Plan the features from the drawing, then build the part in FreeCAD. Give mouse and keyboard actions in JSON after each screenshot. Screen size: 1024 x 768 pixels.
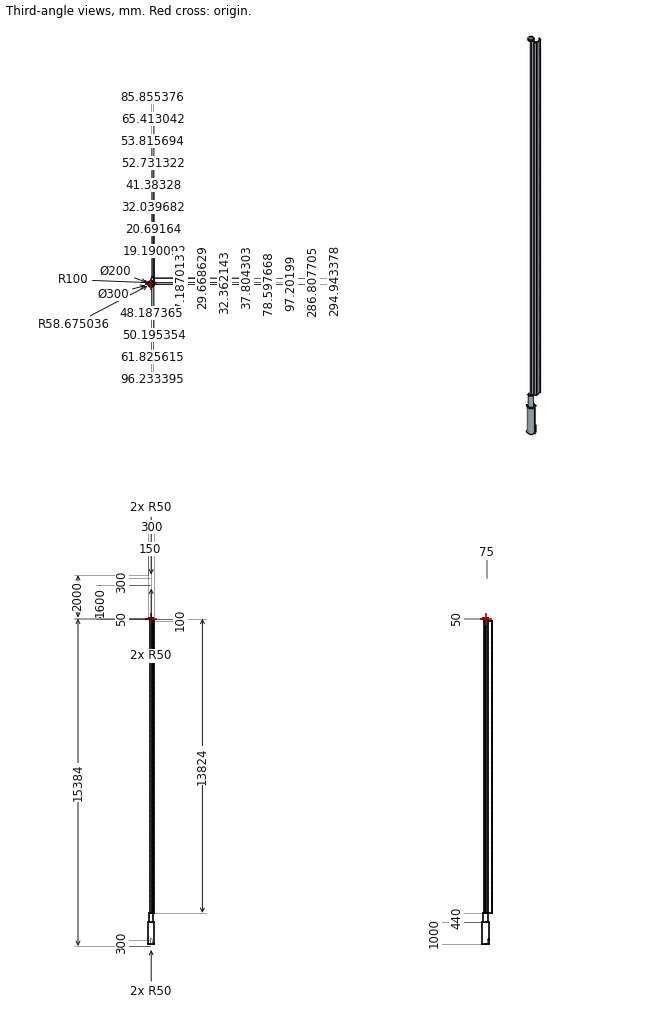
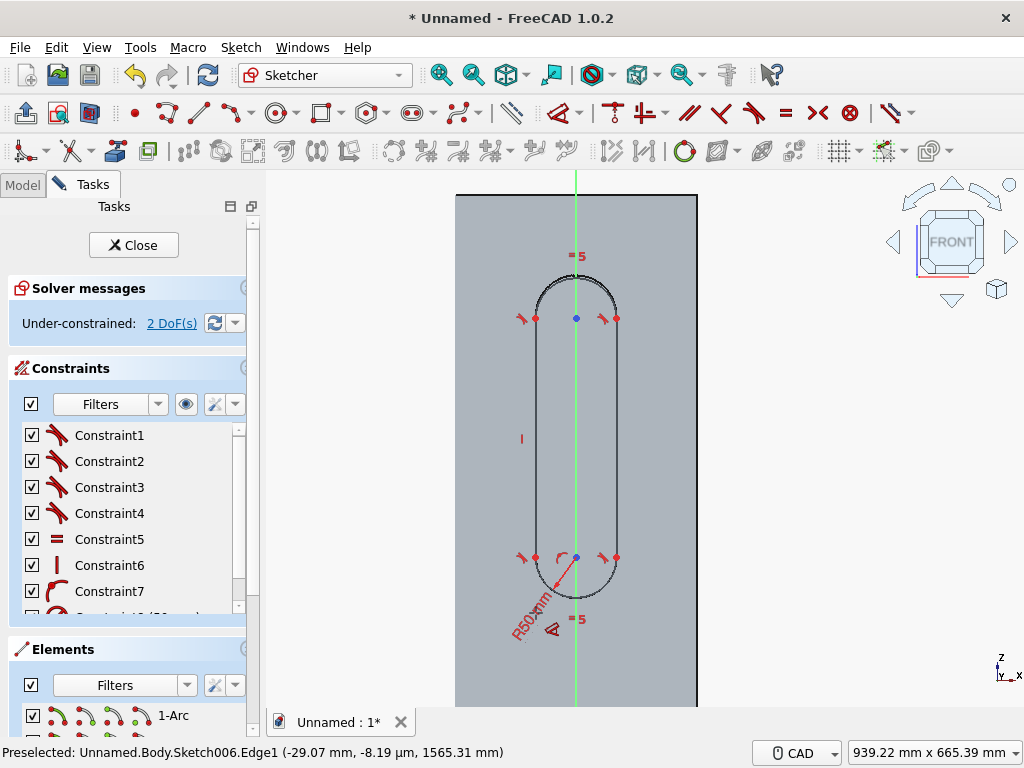
{"action": "left_click", "coordinate": [536, 486]}
{"action": "left_click", "coordinate": [502, 438]}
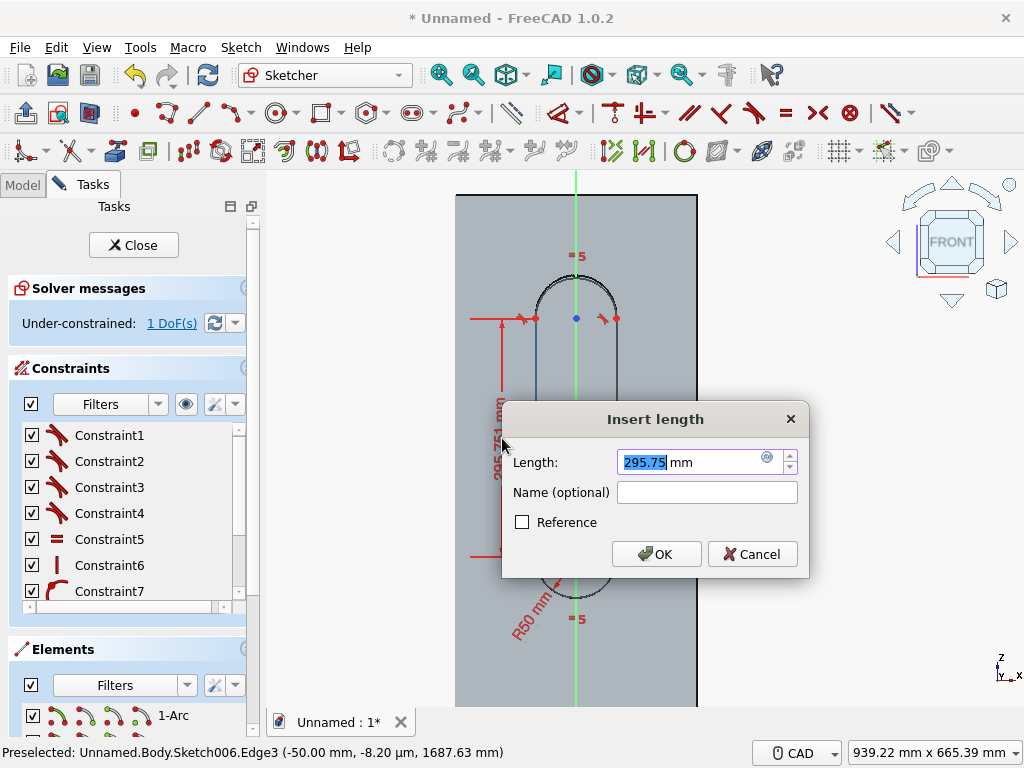
{"action": "type", "text": "300"}
{"action": "key", "text": "Return"}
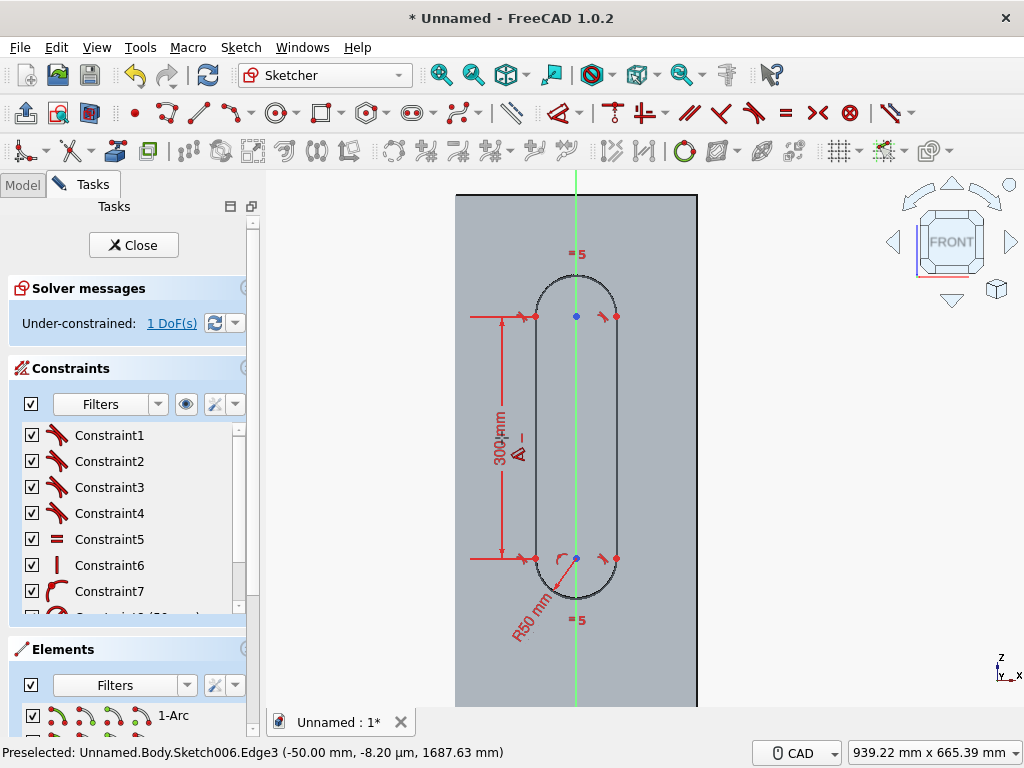
{"action": "left_click", "coordinate": [536, 559]}
{"action": "left_click", "coordinate": [502, 591]}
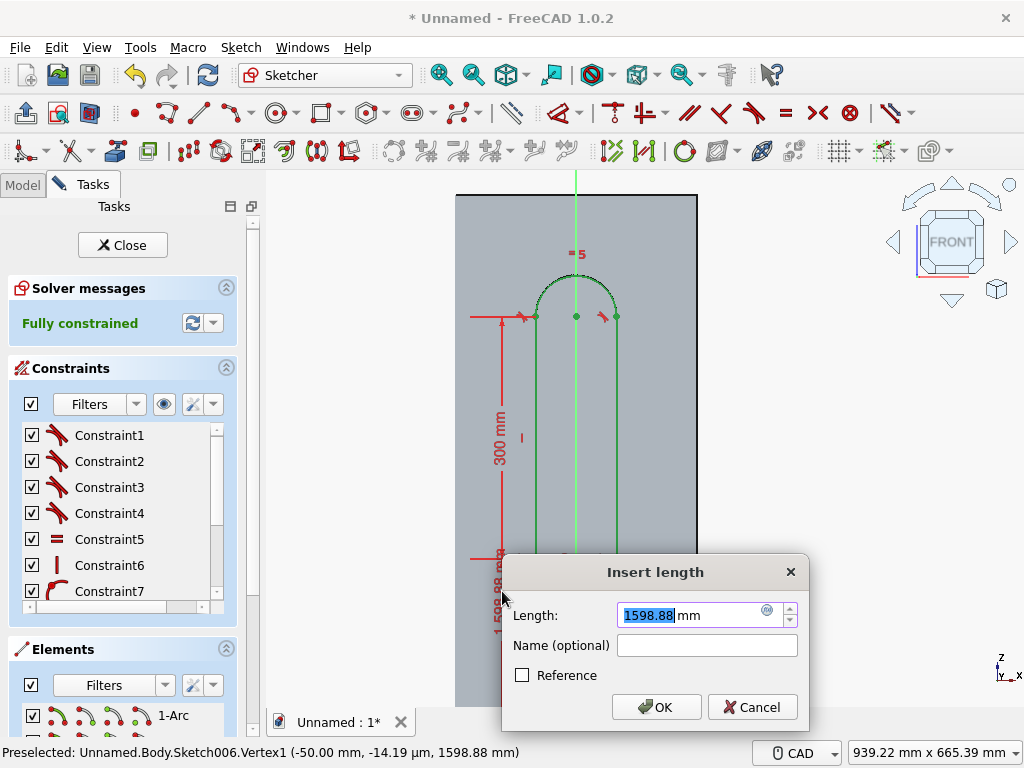
{"action": "type", "text": "1600"}
{"action": "key", "text": "Return"}
{"action": "key", "text": "Escape"}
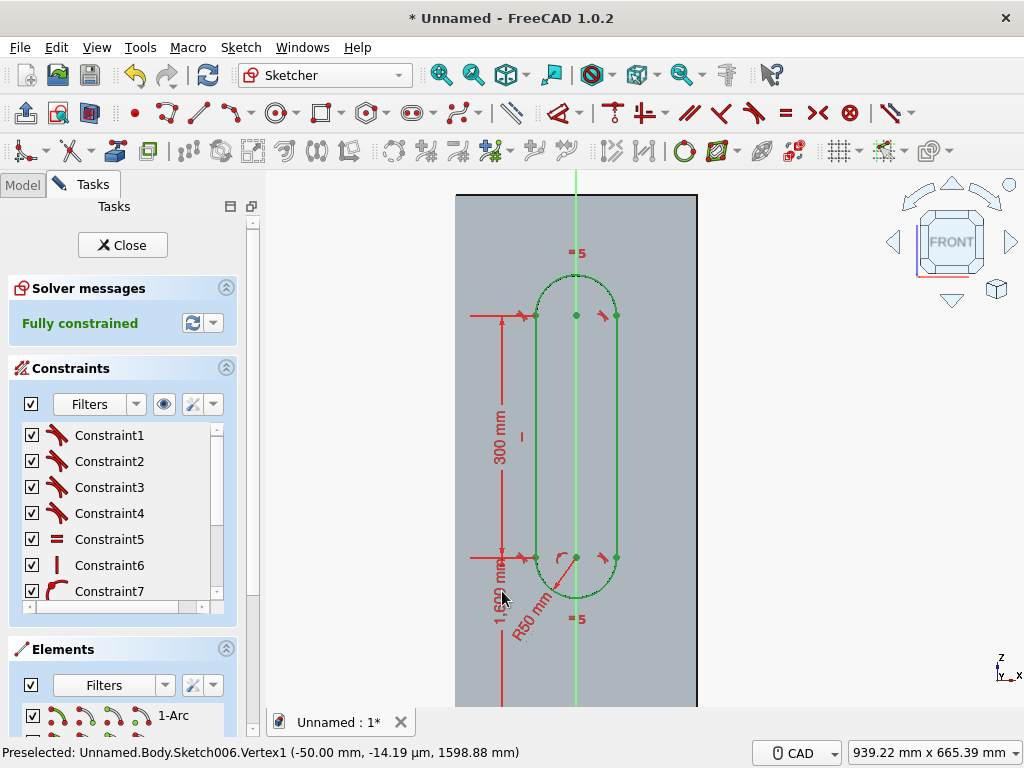
{"action": "left_click", "coordinate": [123, 245]}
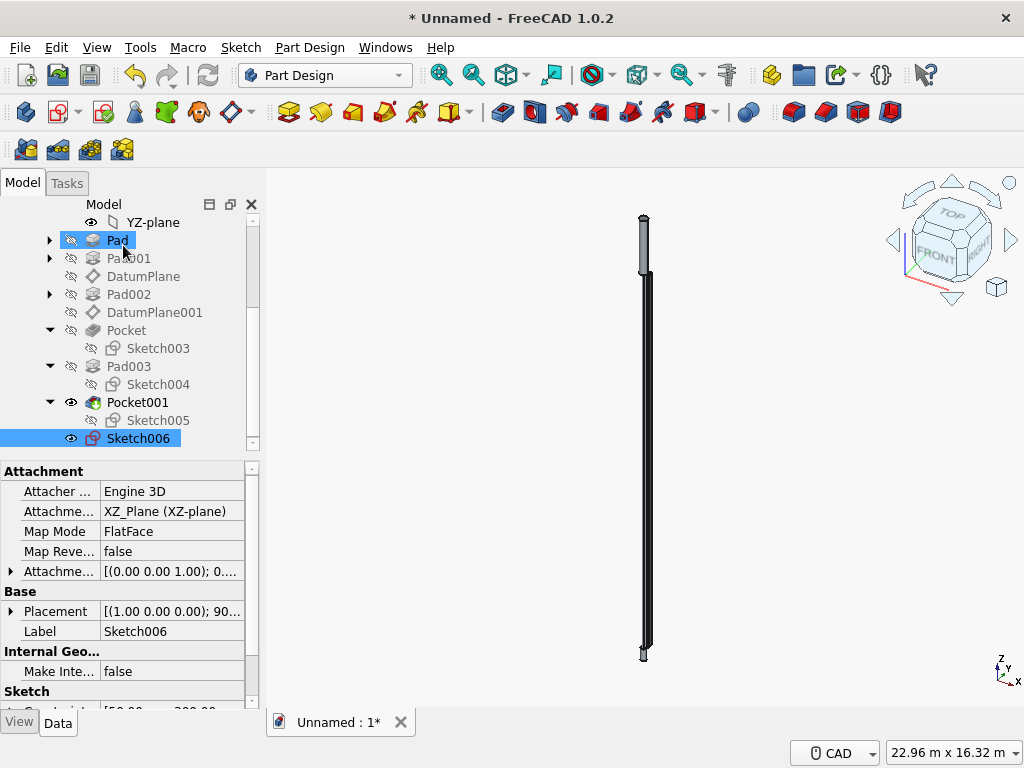
{"action": "left_click", "coordinate": [290, 112]}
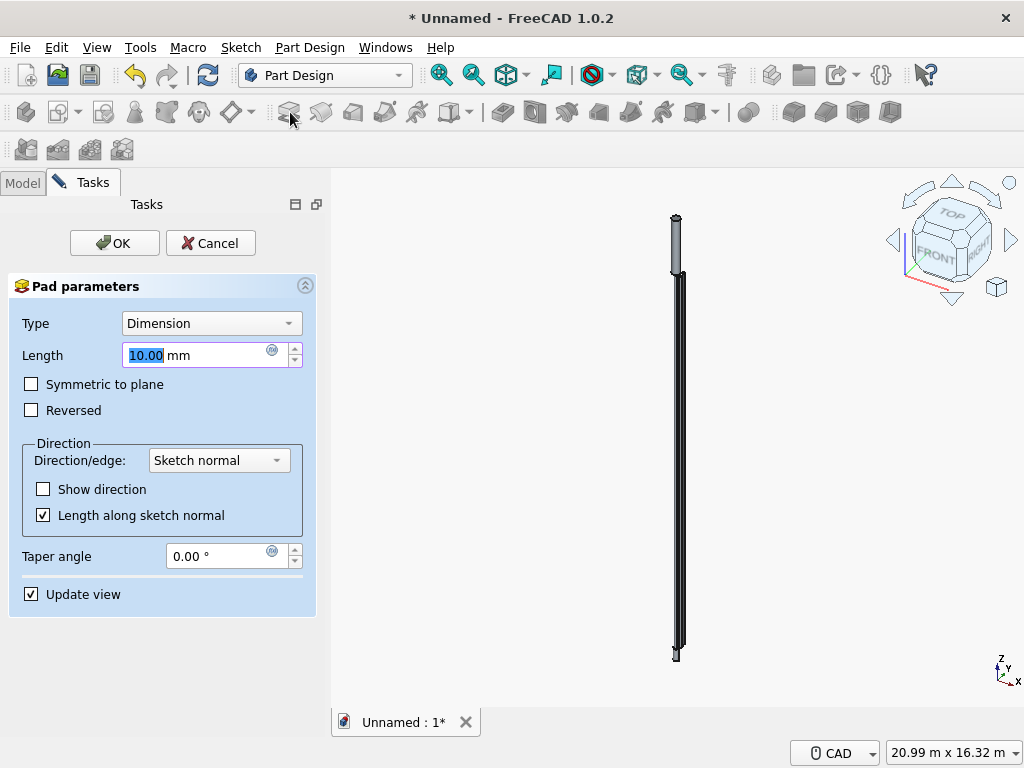
{"action": "type", "text": "75"}
{"action": "key", "text": "Tab"}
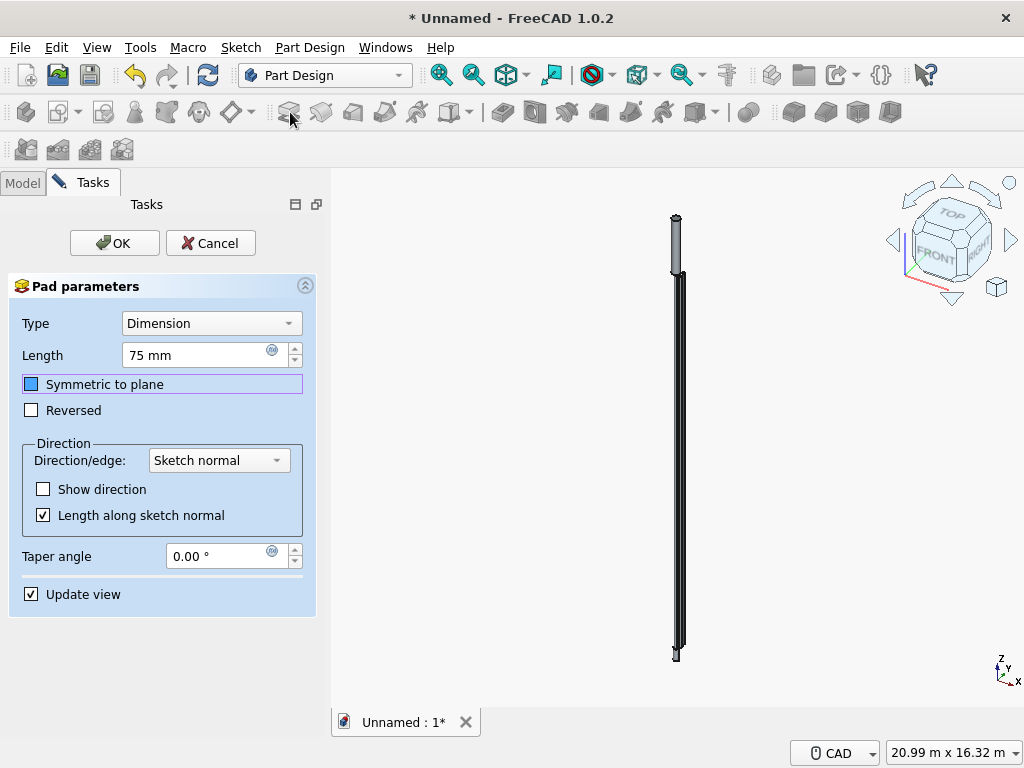
{"action": "left_click", "coordinate": [30, 410]}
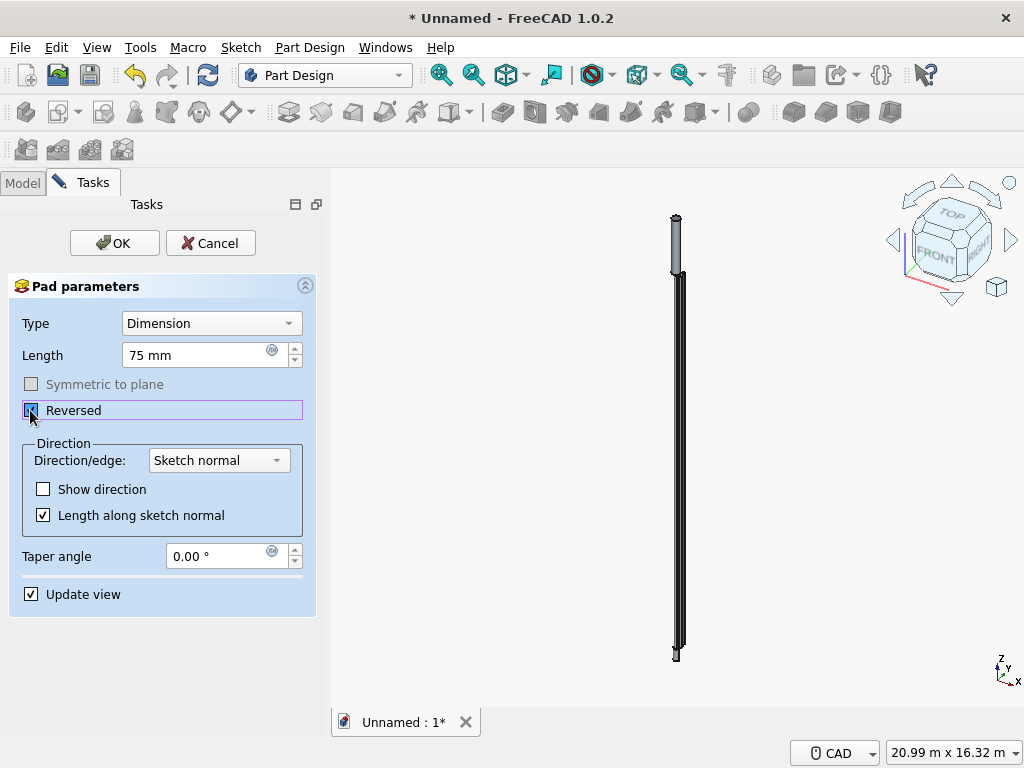
{"action": "left_click", "coordinate": [115, 243]}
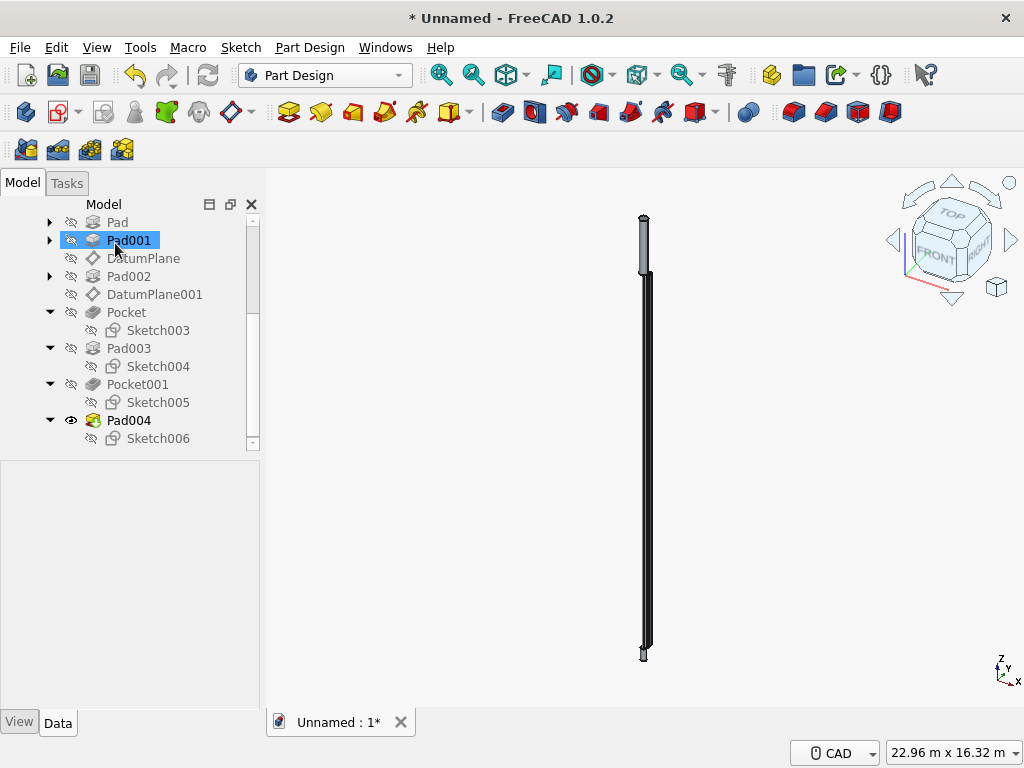
{"action": "scroll", "coordinate": [140, 326], "scroll_direction": "down", "scroll_amount": 3}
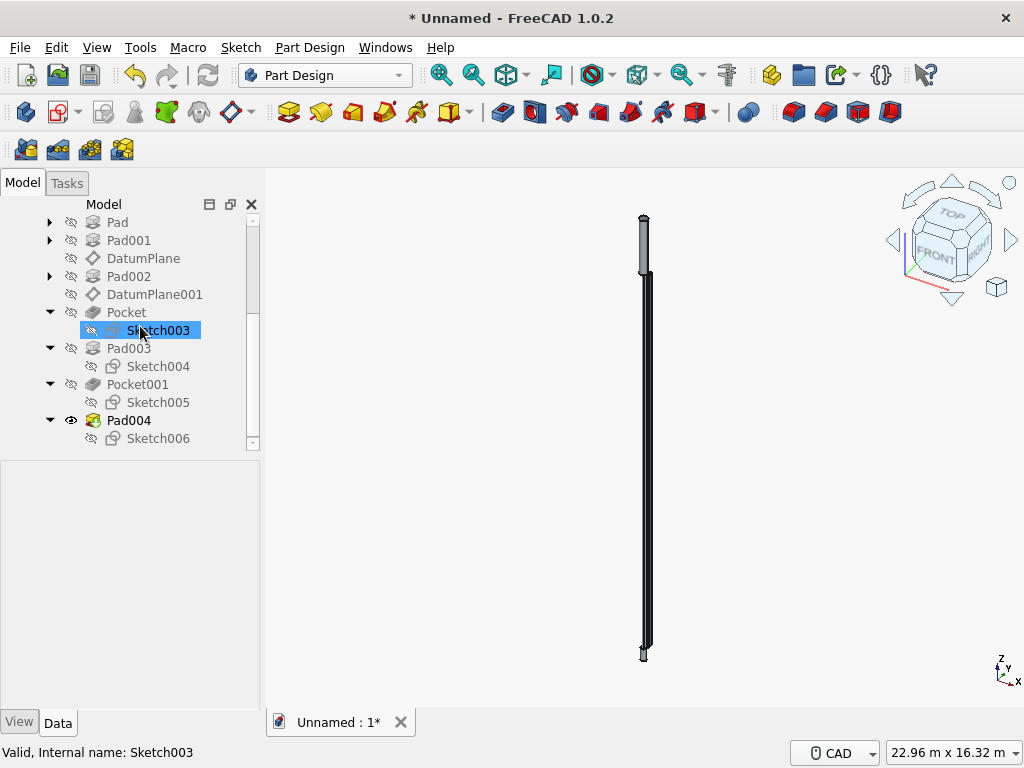
{"action": "scroll", "coordinate": [140, 326], "scroll_direction": "up", "scroll_amount": 15}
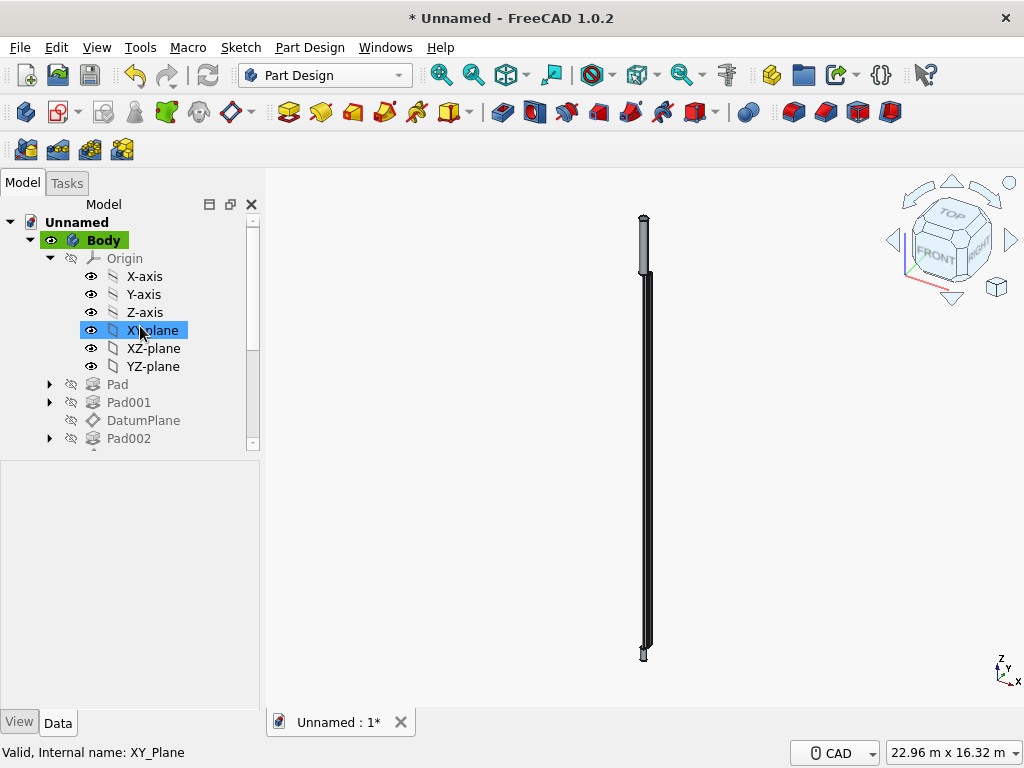
{"action": "left_click", "coordinate": [136, 330]}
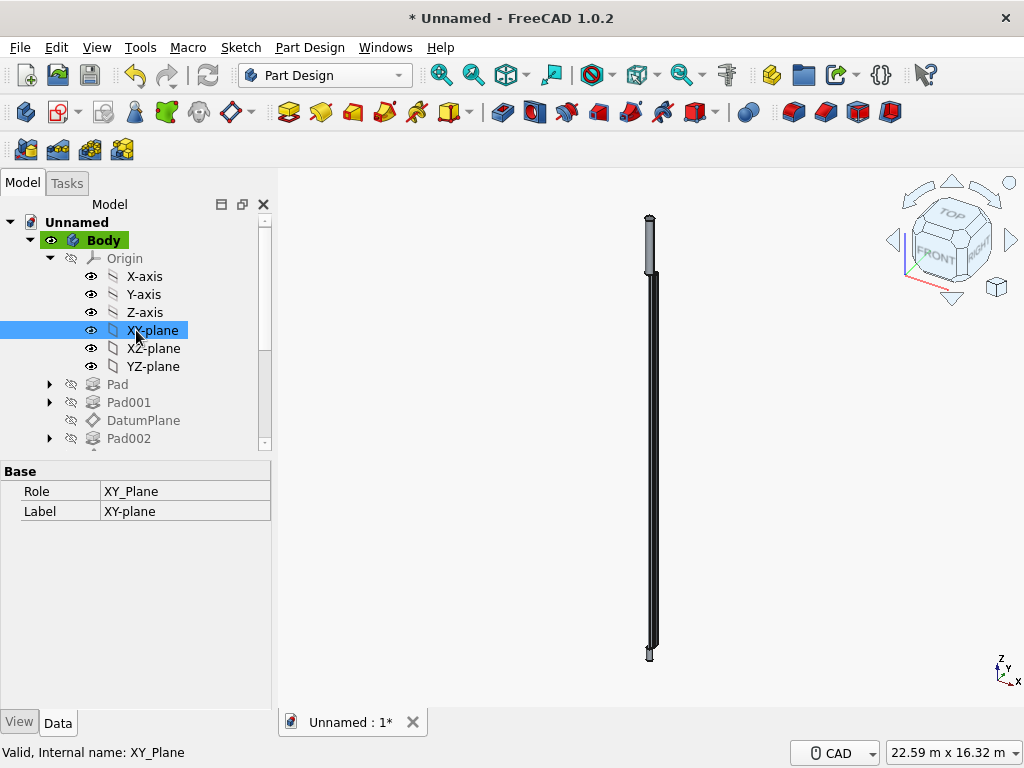
{"action": "left_click", "coordinate": [232, 112]}